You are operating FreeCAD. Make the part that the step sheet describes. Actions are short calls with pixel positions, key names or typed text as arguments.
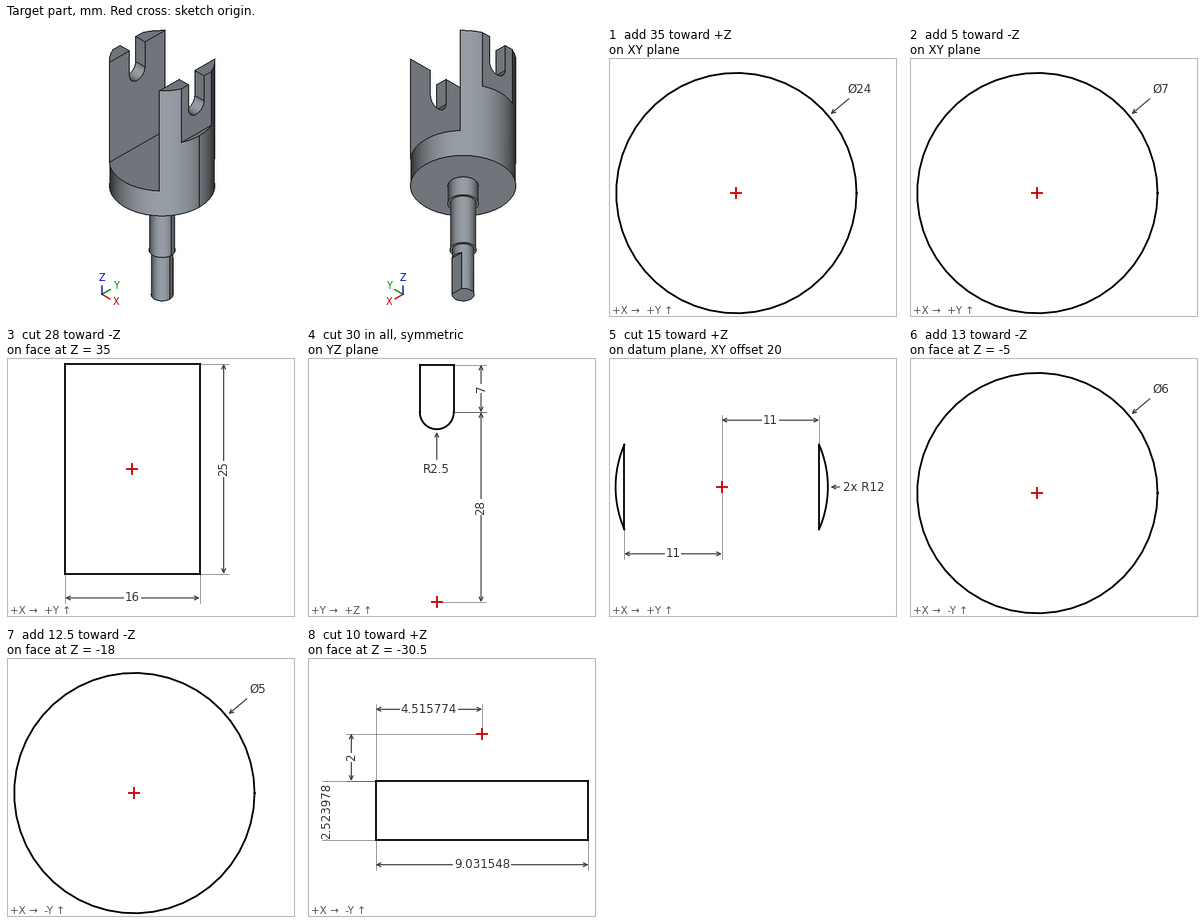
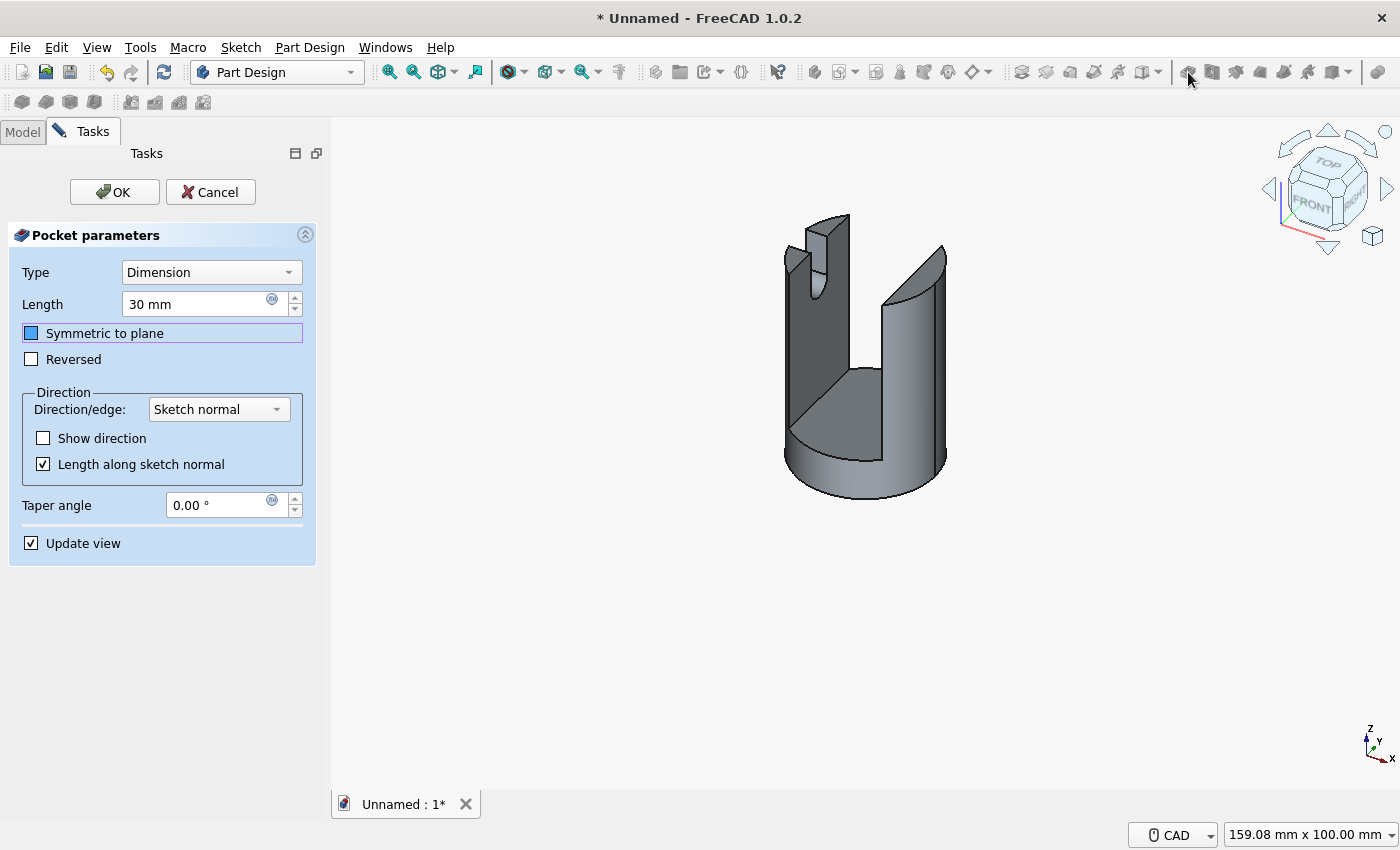
click(30, 333)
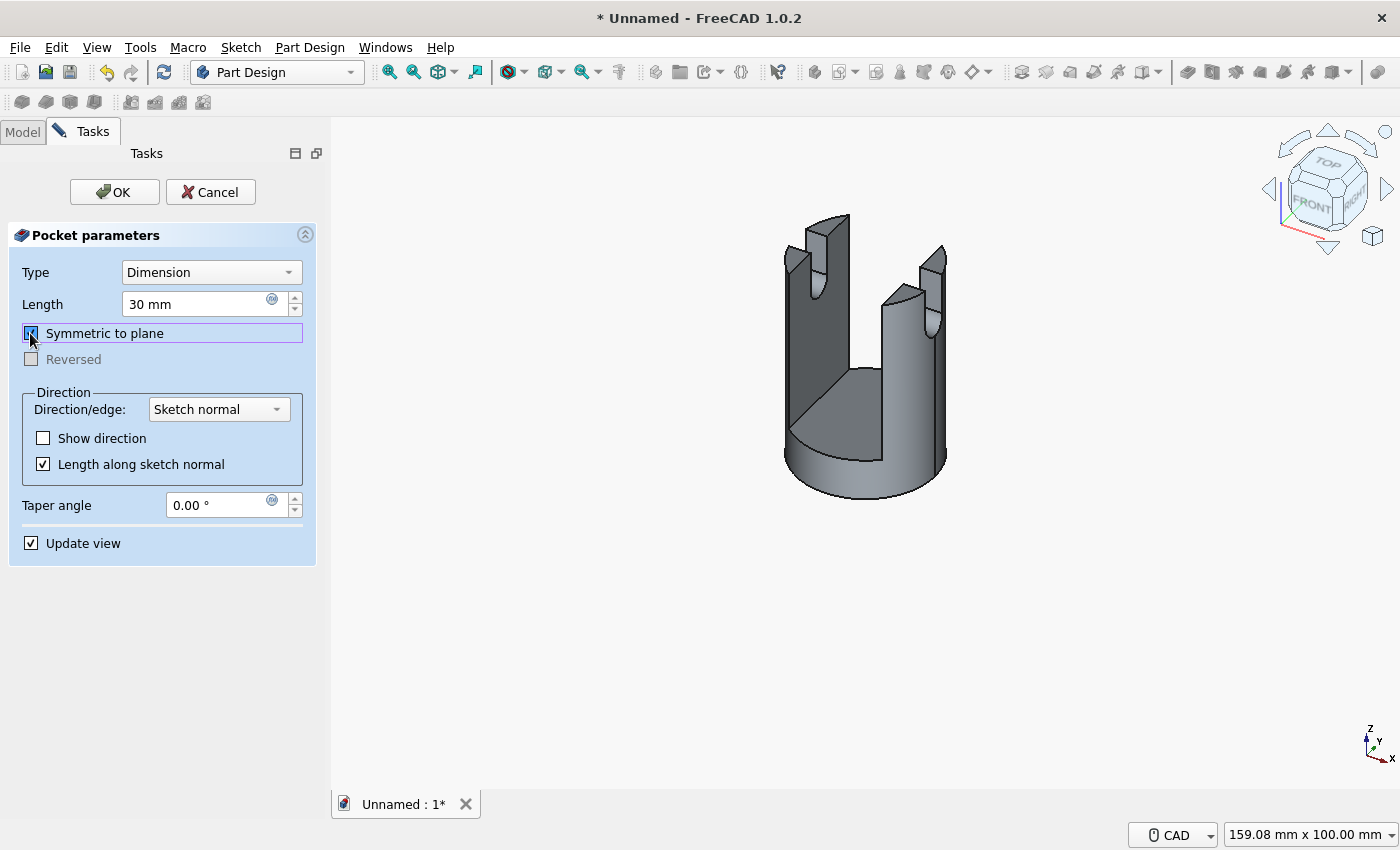
click(115, 192)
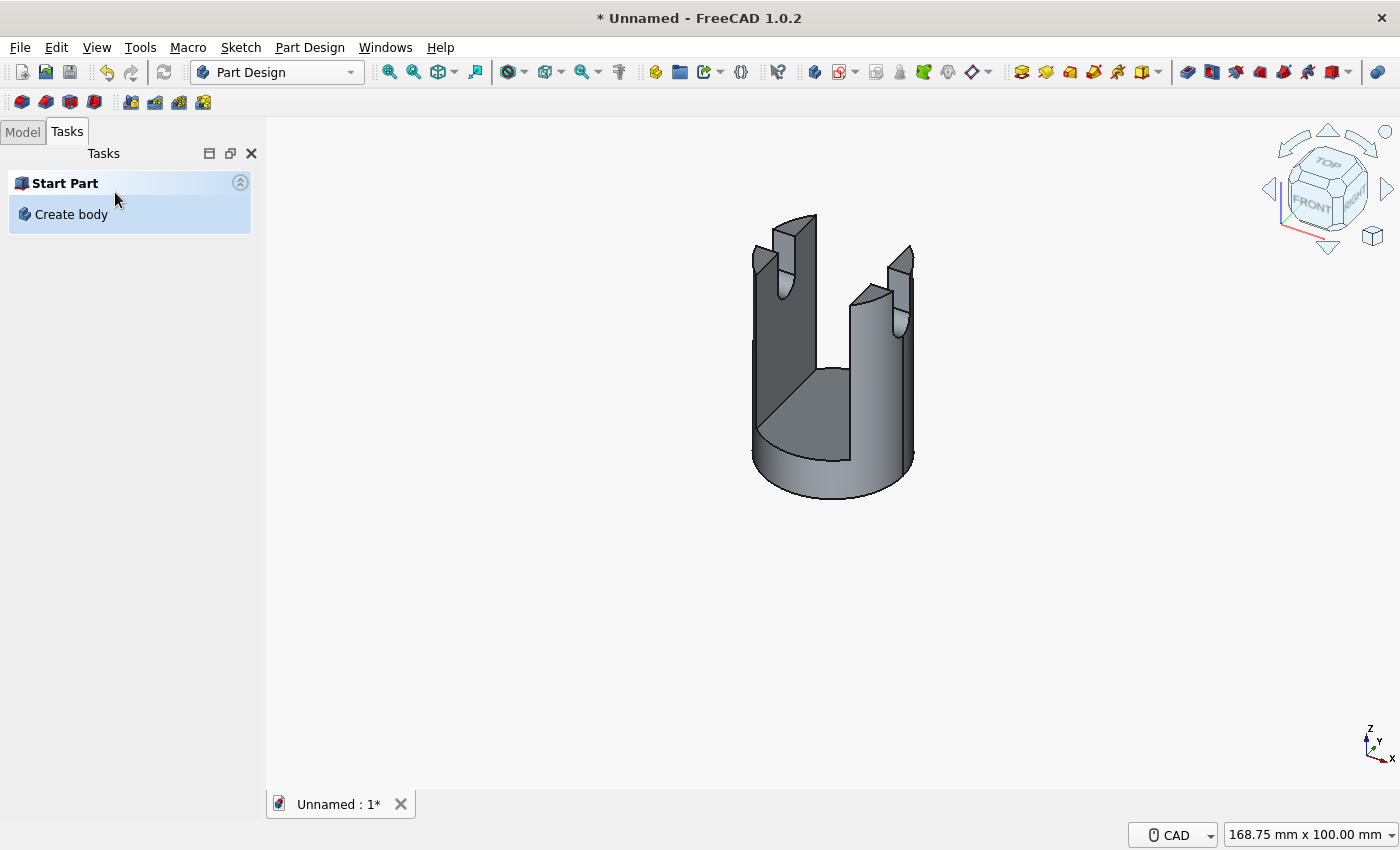
click(23, 131)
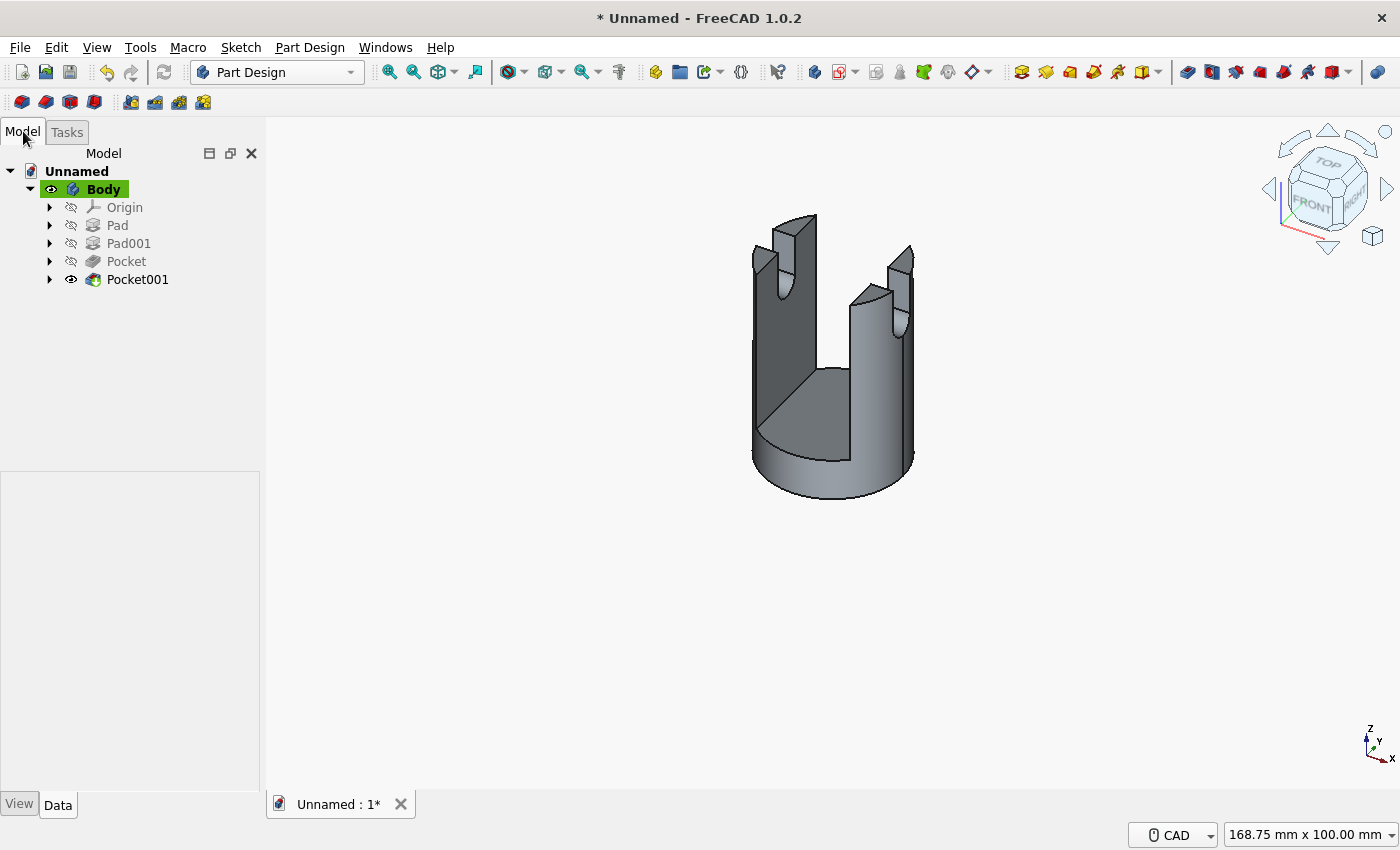
click(50, 207)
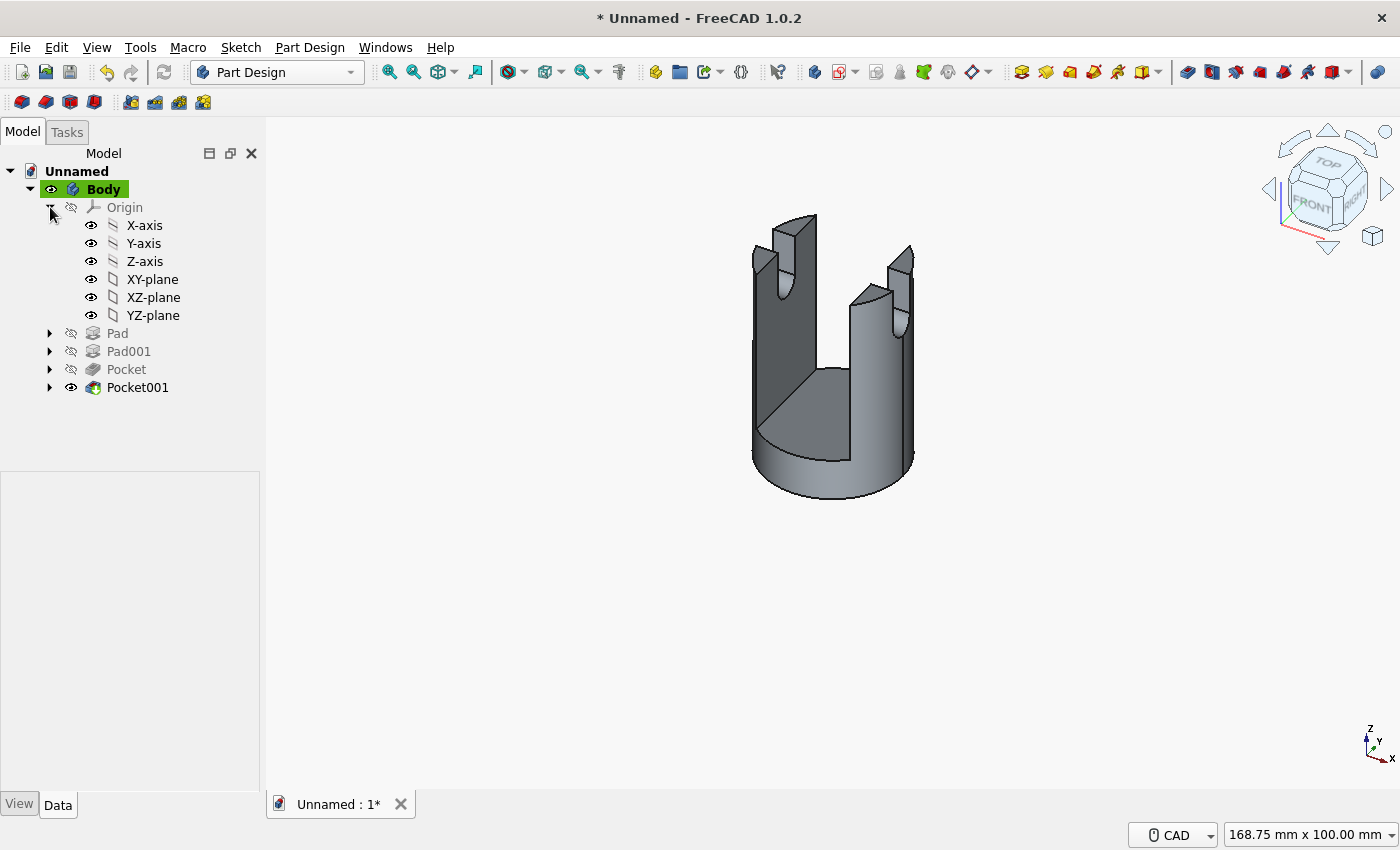
click(136, 279)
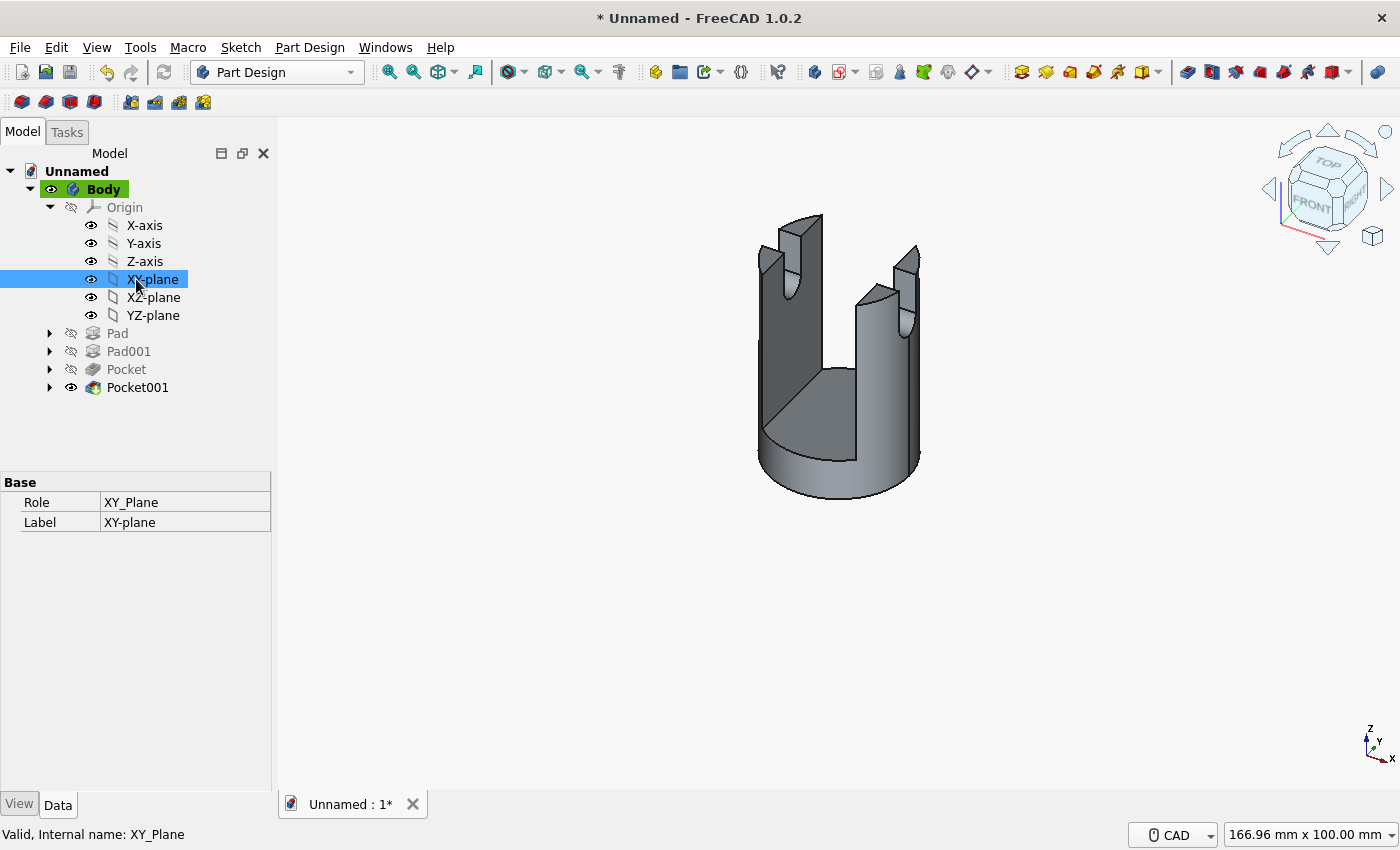
click(972, 72)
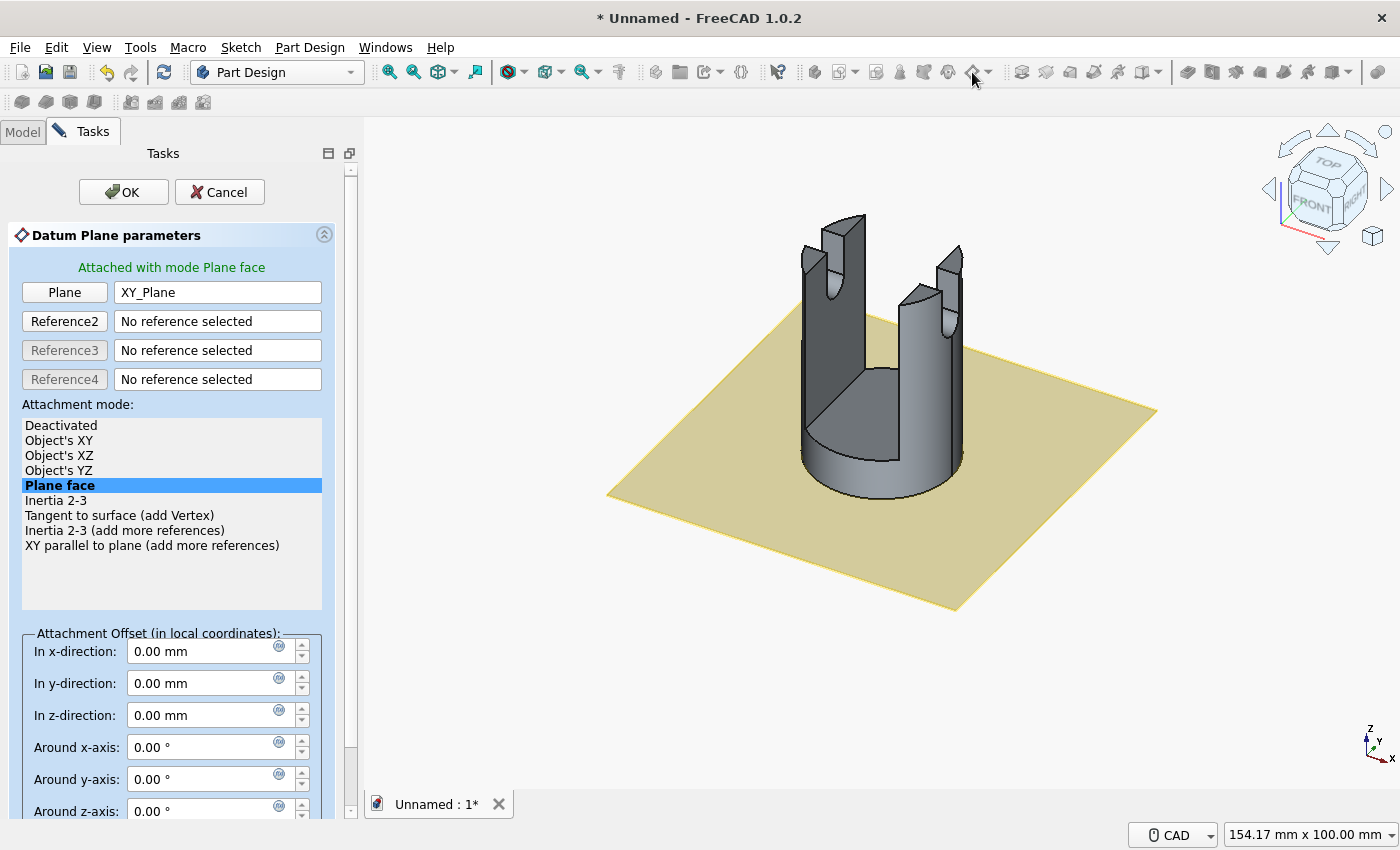
triple_click(210, 715)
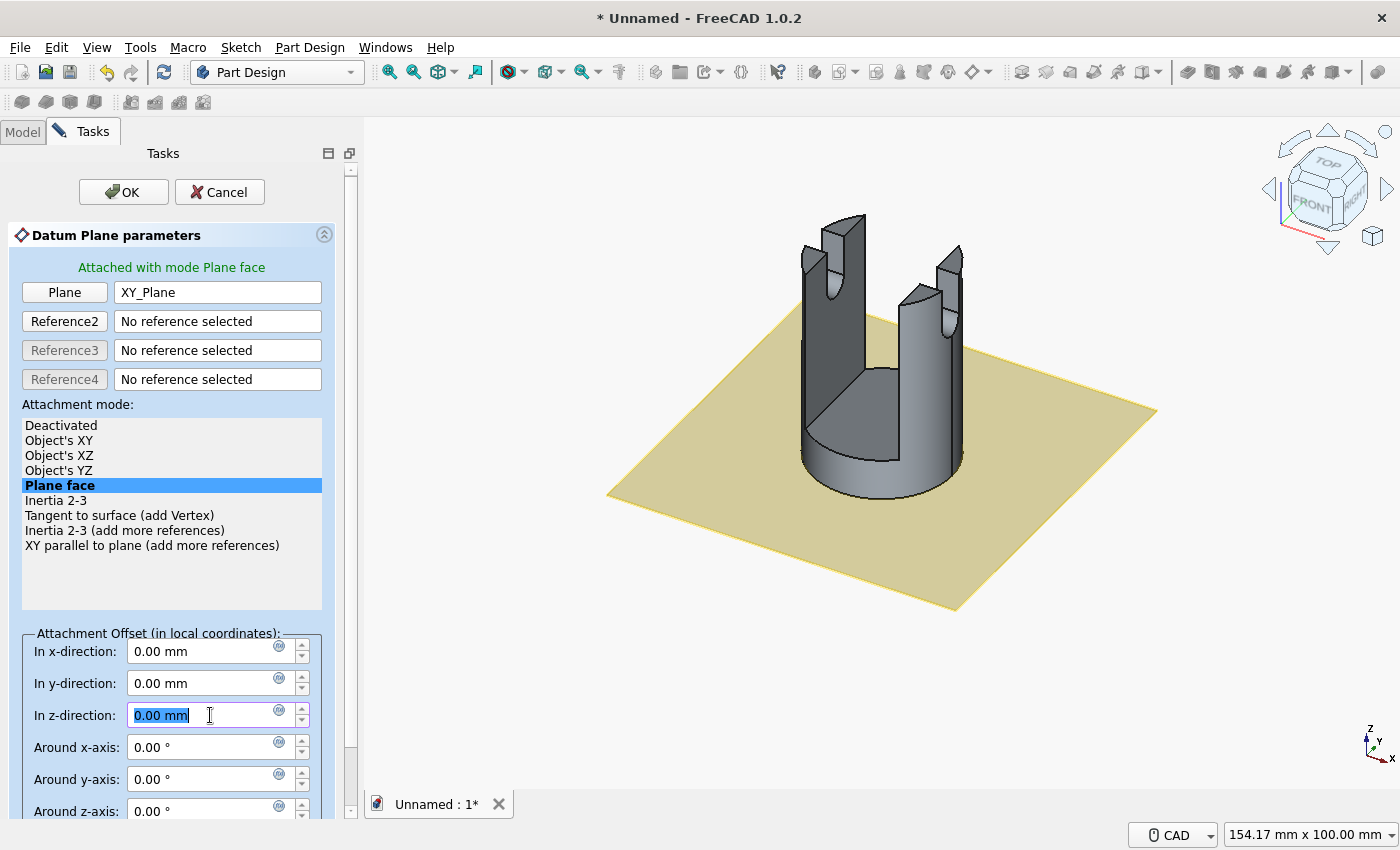
text(20)
key(Tab)